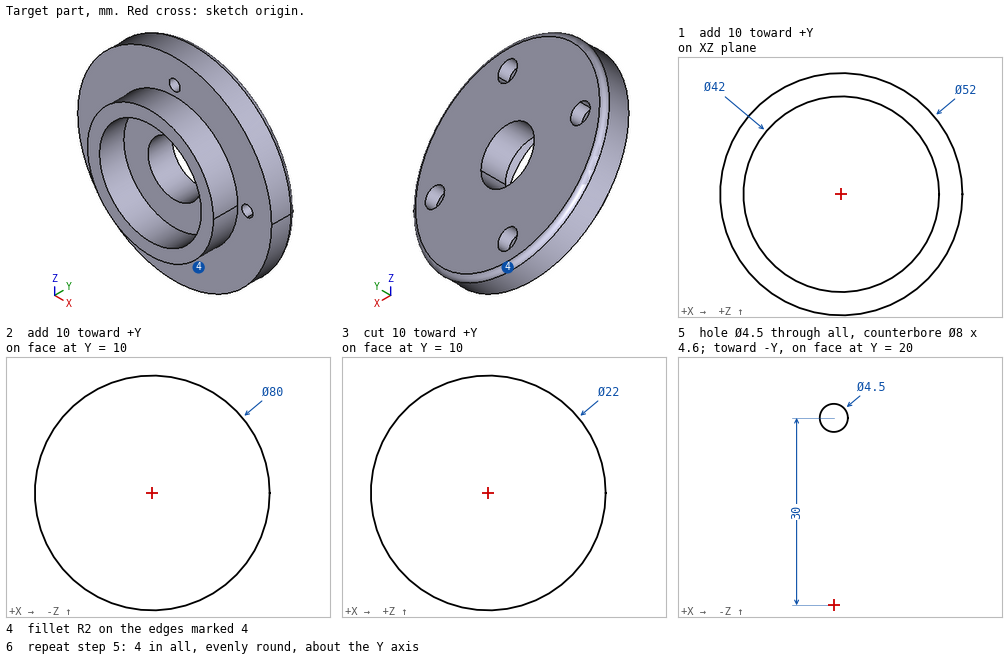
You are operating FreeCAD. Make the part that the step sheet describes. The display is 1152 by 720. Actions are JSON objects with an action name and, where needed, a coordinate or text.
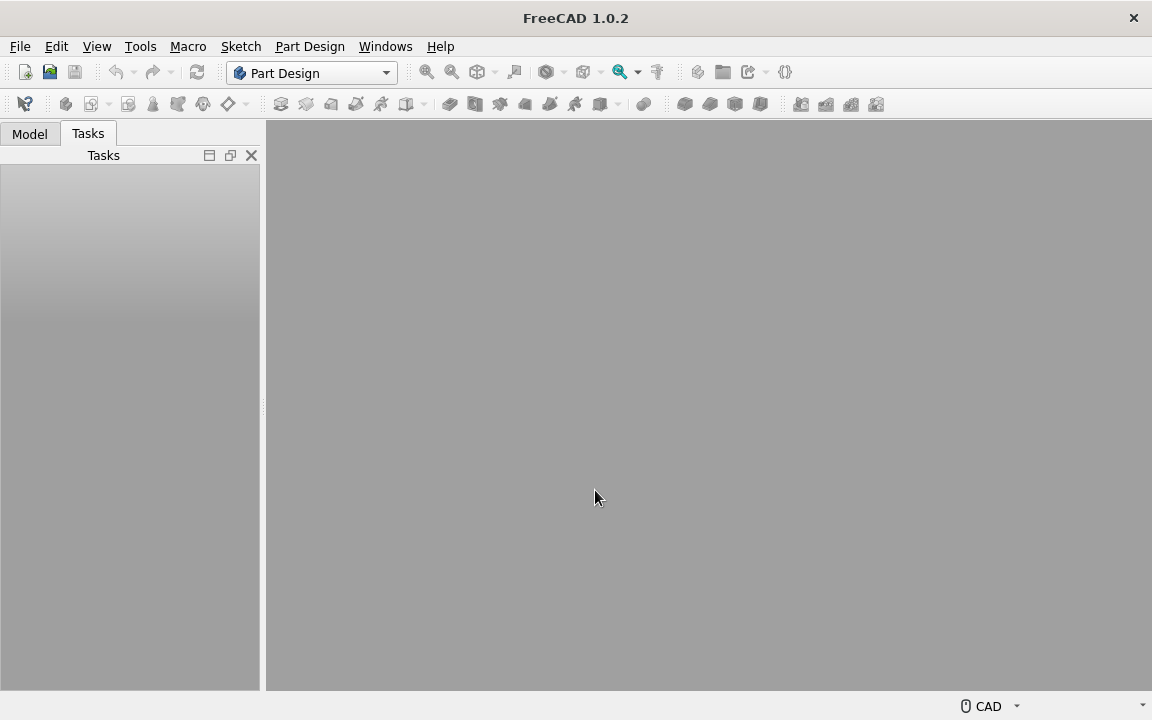
{"action": "left_click", "coordinate": [25, 72]}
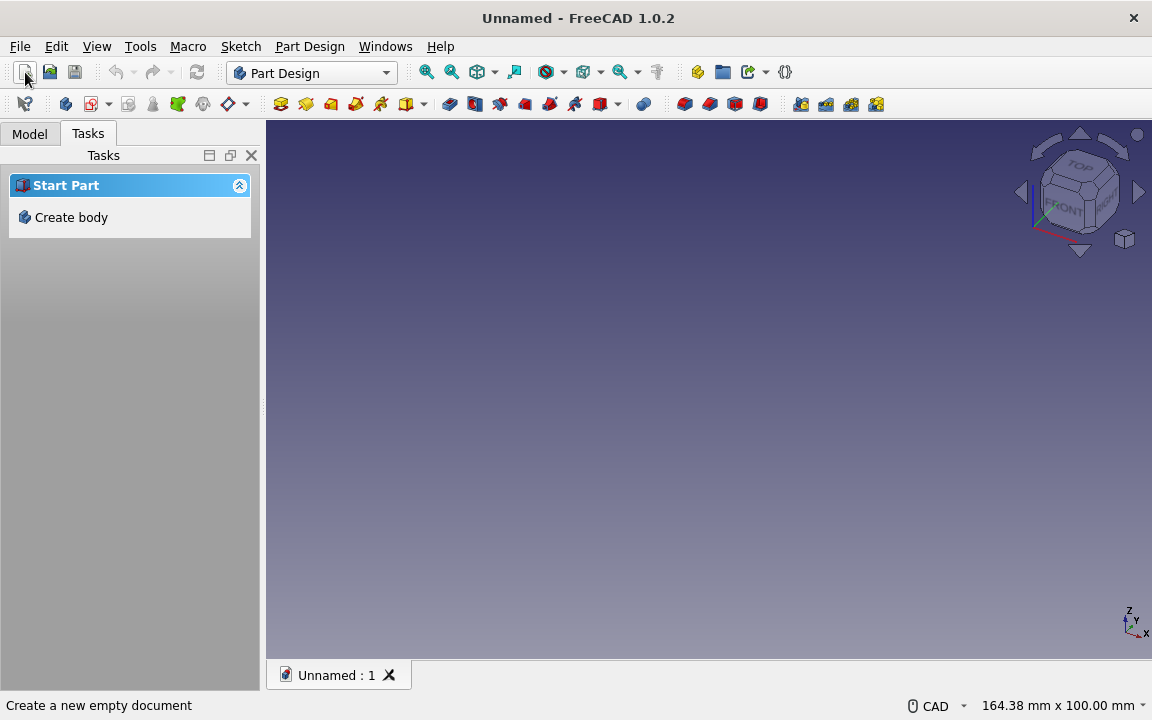
{"action": "left_click", "coordinate": [90, 104]}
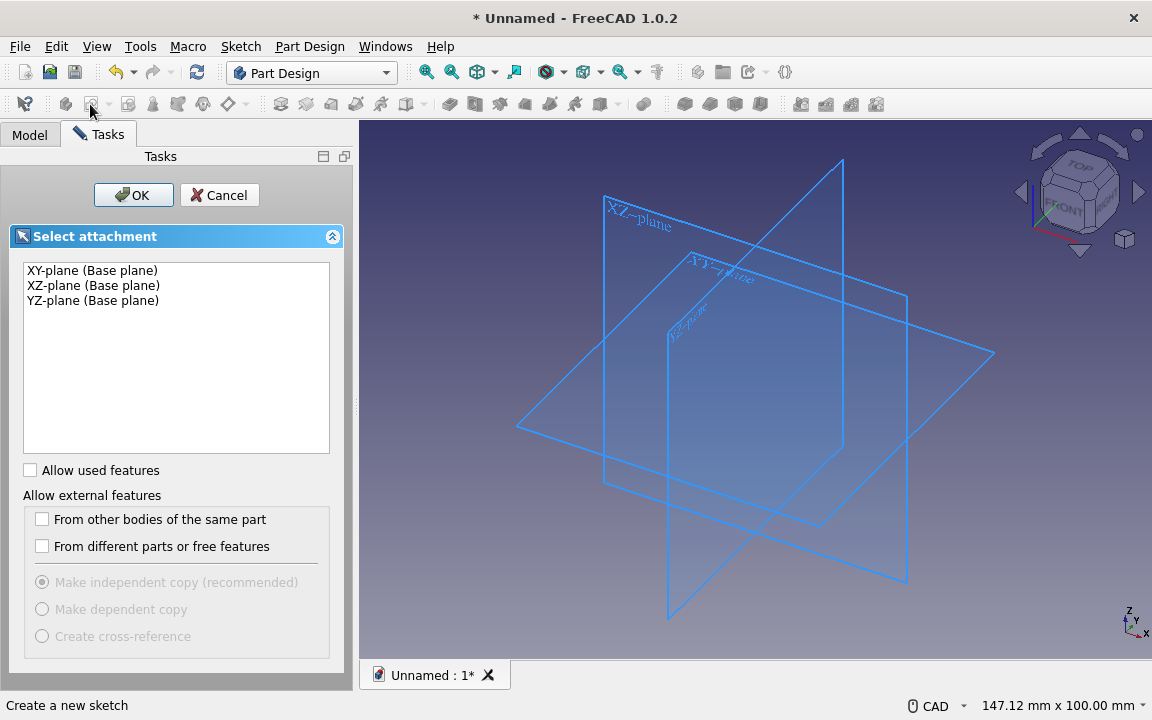
{"action": "left_click", "coordinate": [84, 286]}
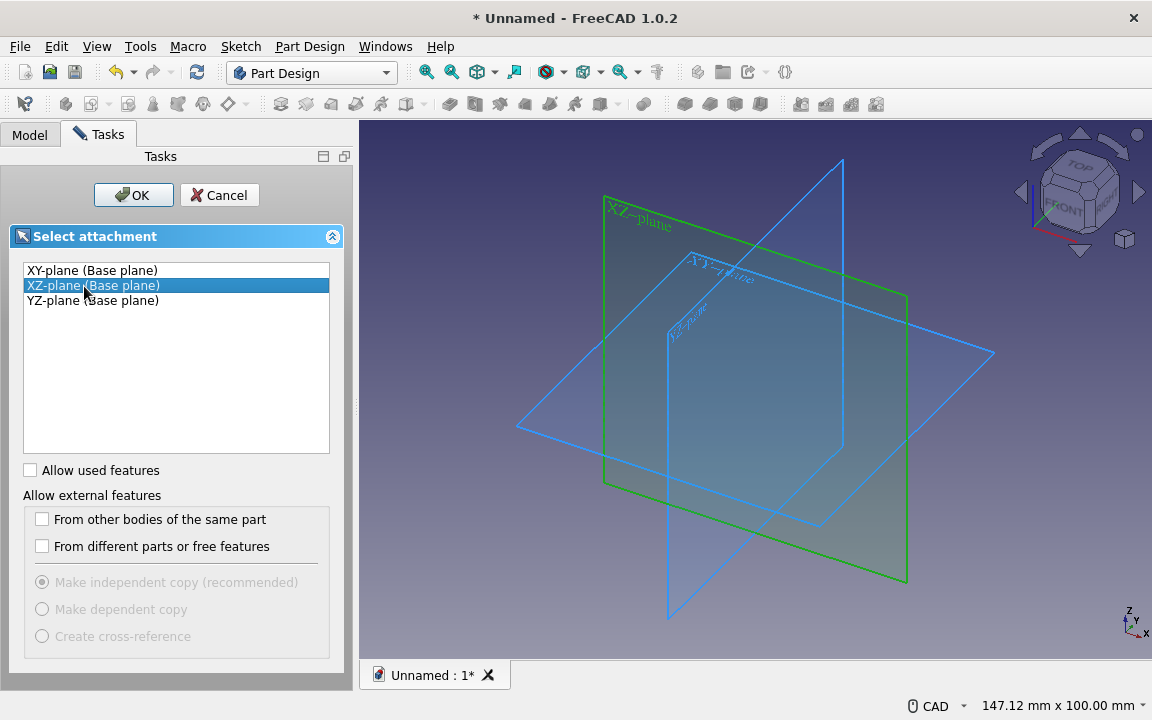
{"action": "left_click", "coordinate": [134, 195]}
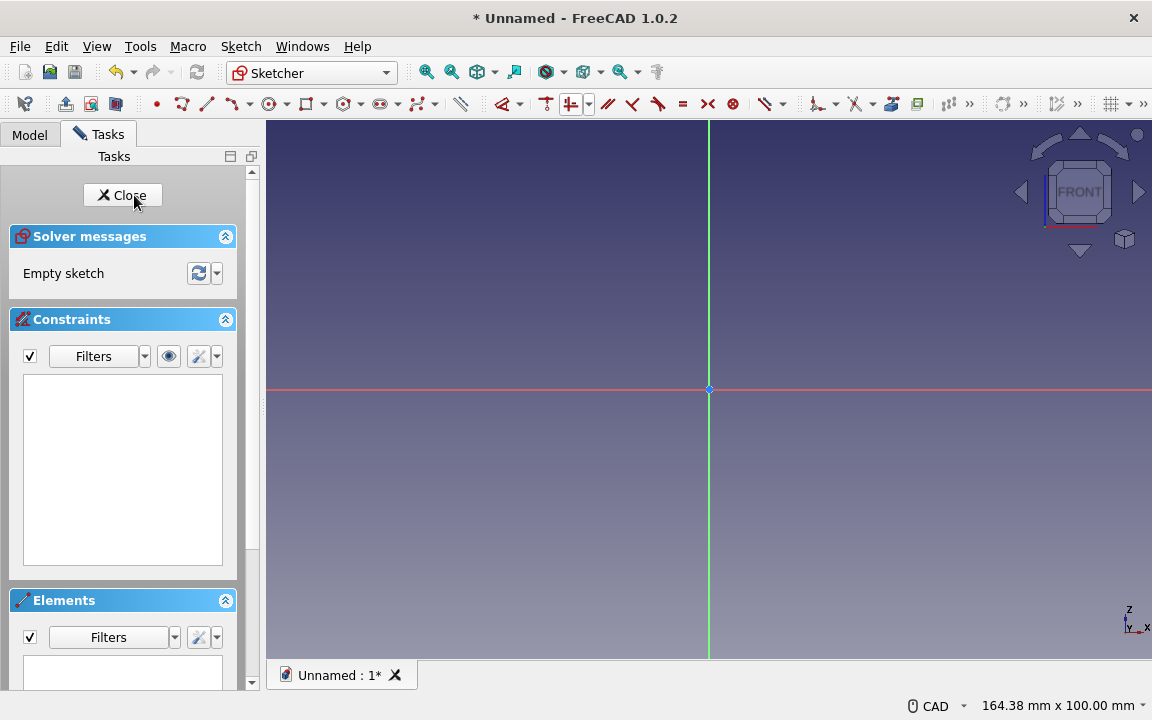
{"action": "left_click", "coordinate": [268, 104]}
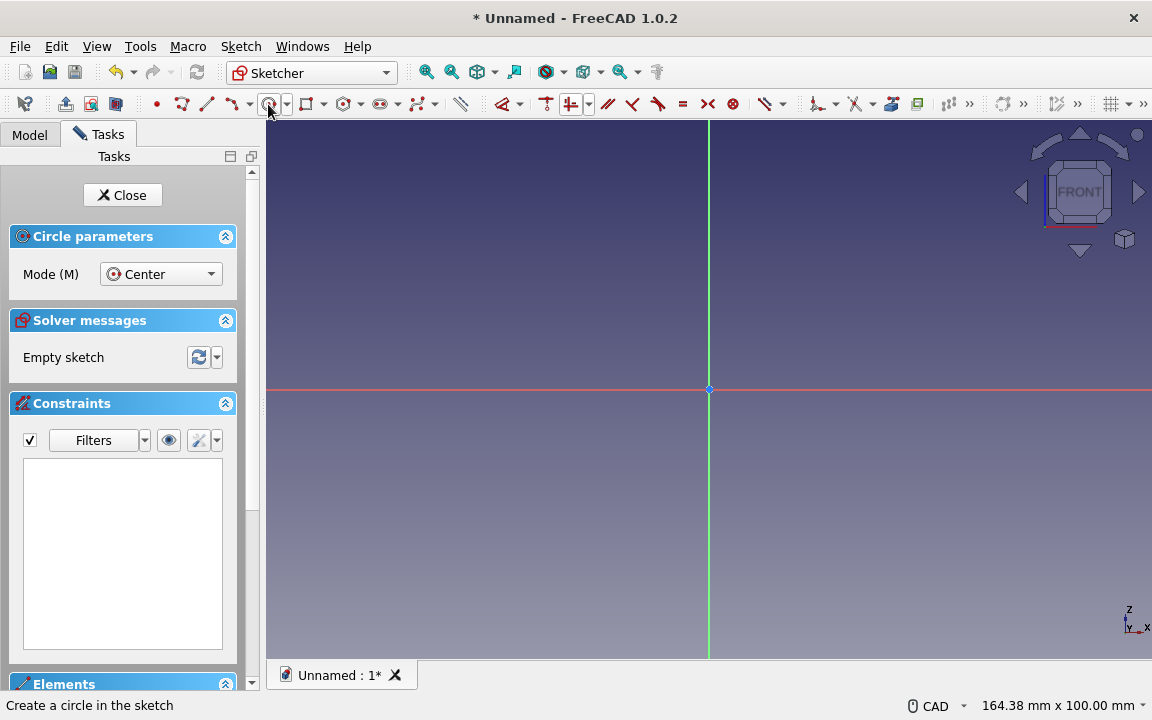
{"action": "left_click", "coordinate": [709, 390]}
{"action": "left_click", "coordinate": [808, 290]}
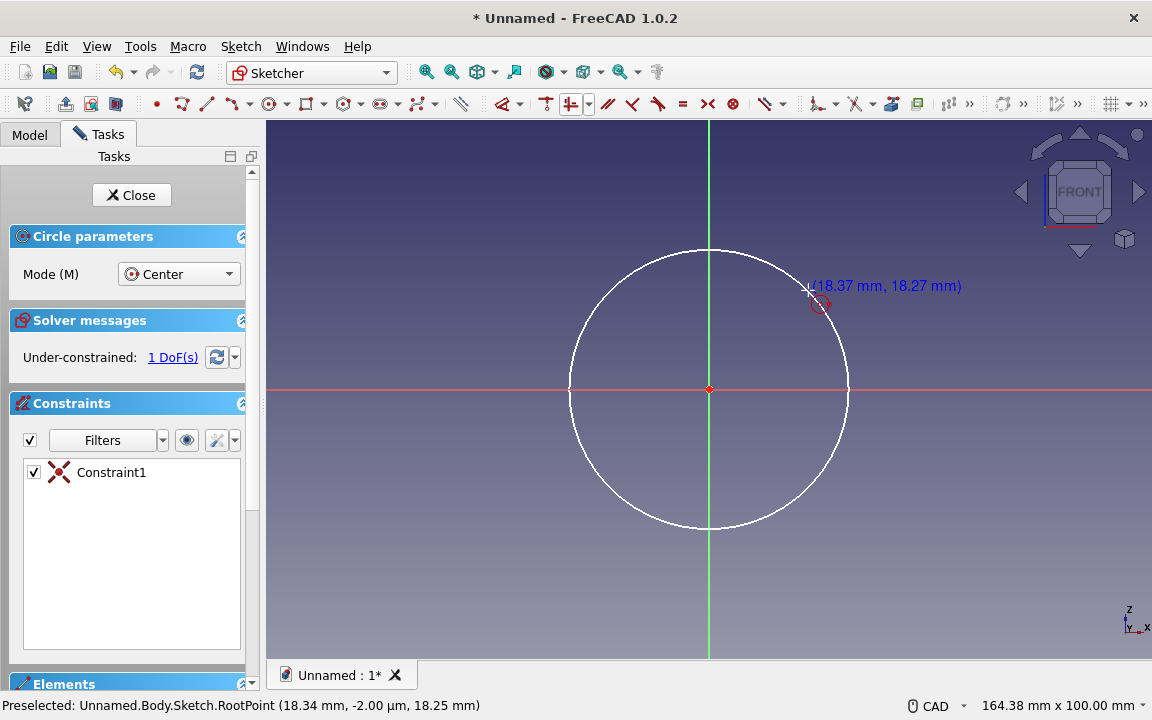
{"action": "left_click", "coordinate": [709, 390]}
{"action": "left_click", "coordinate": [789, 309]}
{"action": "key", "text": "Escape"}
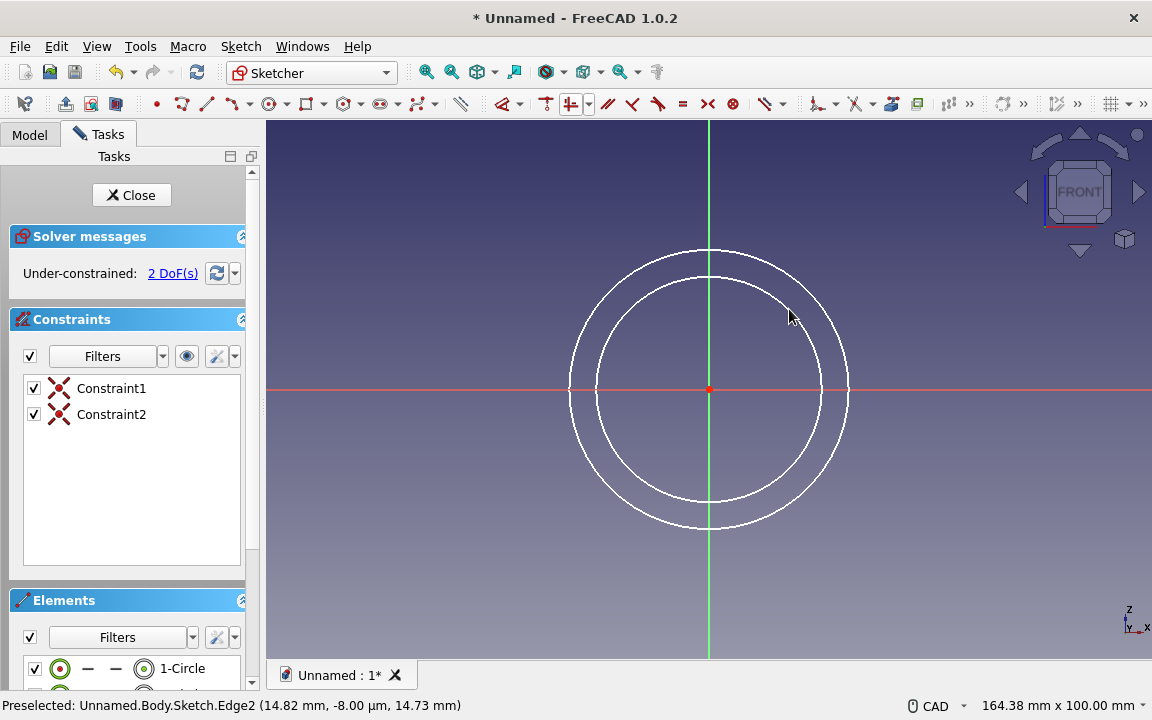
{"action": "left_click", "coordinate": [502, 104]}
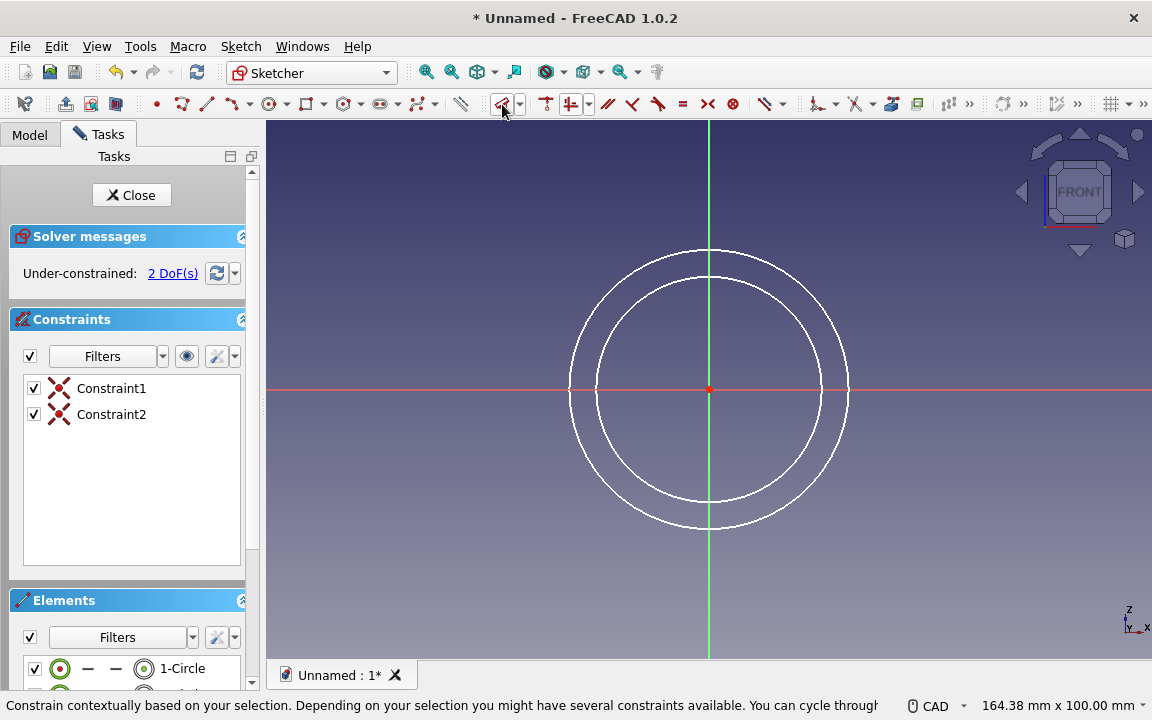
{"action": "left_click", "coordinate": [807, 290]}
{"action": "left_click", "coordinate": [829, 267]}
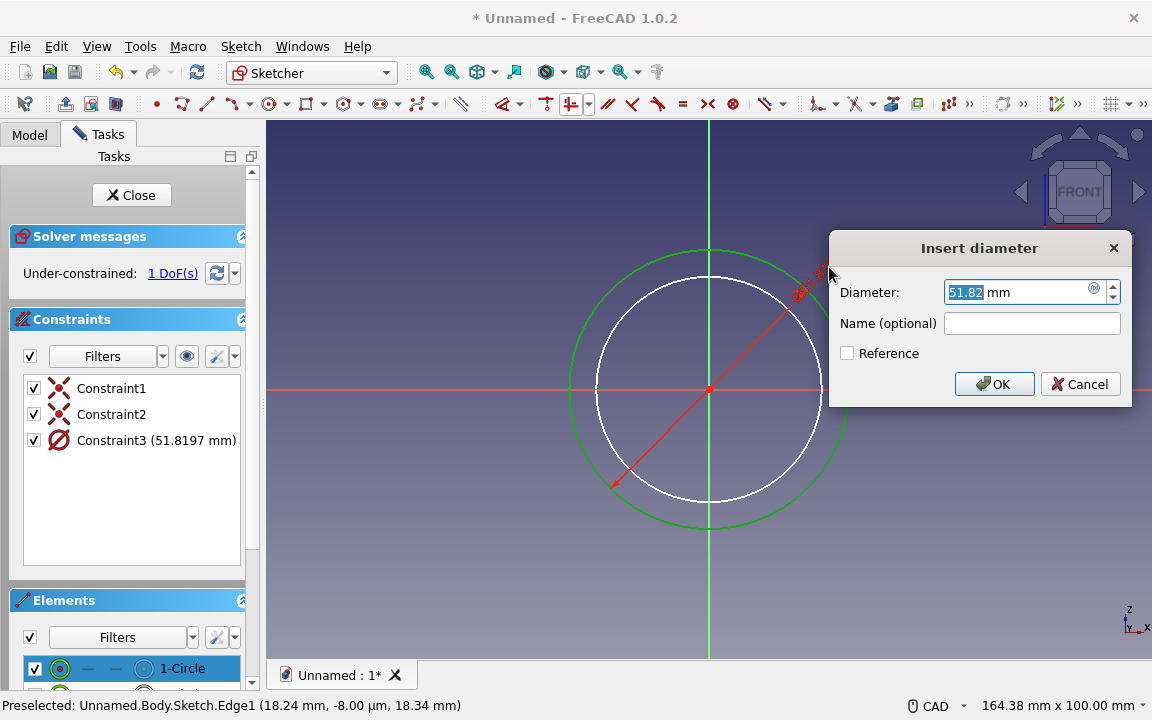
{"action": "type", "text": "52"}
{"action": "key", "text": "Return"}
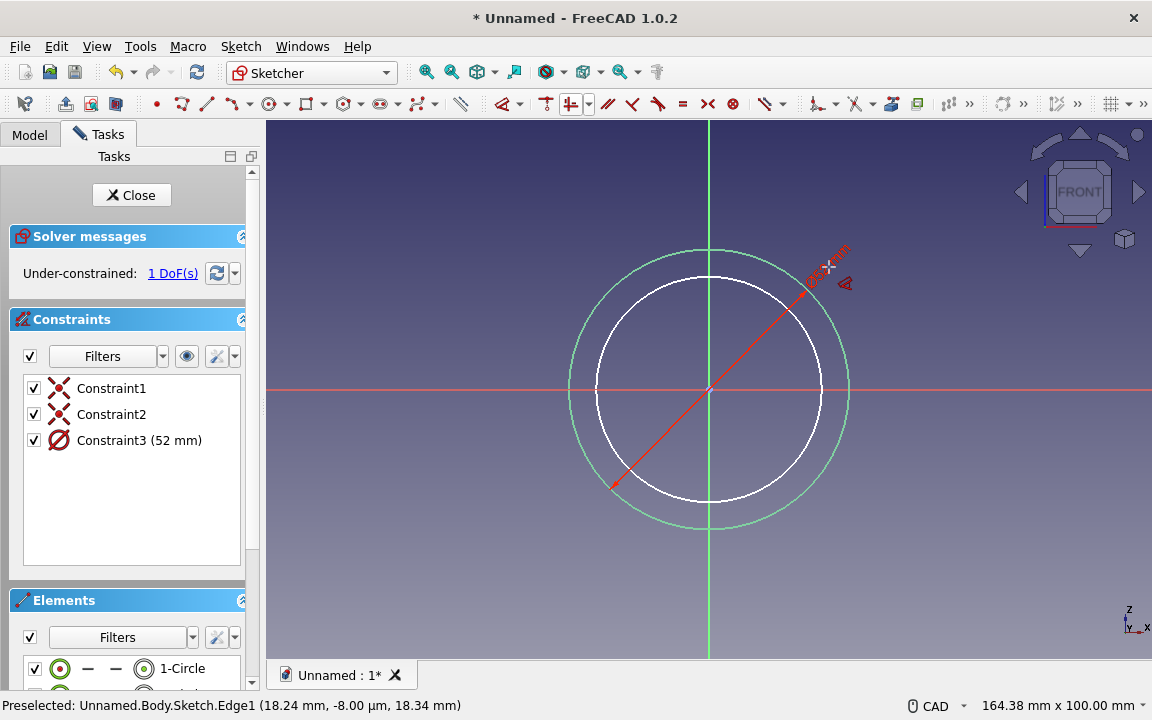
{"action": "left_click", "coordinate": [789, 310]}
{"action": "left_click", "coordinate": [870, 343]}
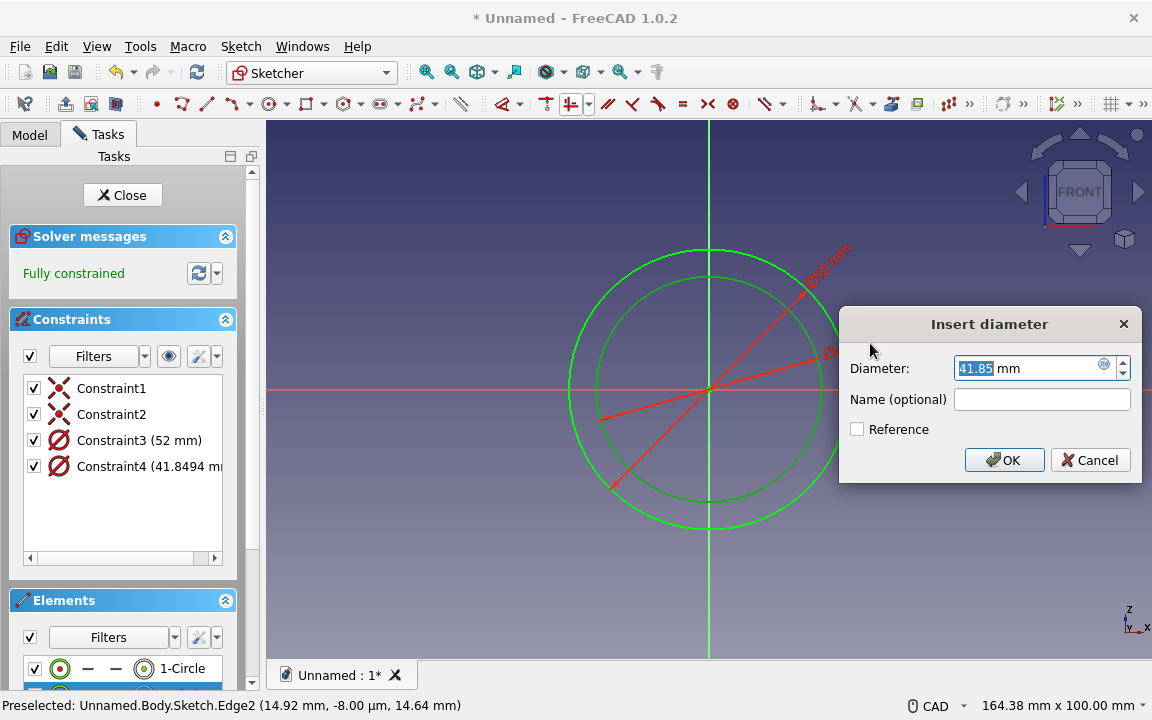
{"action": "type", "text": "42"}
{"action": "key", "text": "Return"}
{"action": "key", "text": "Escape"}